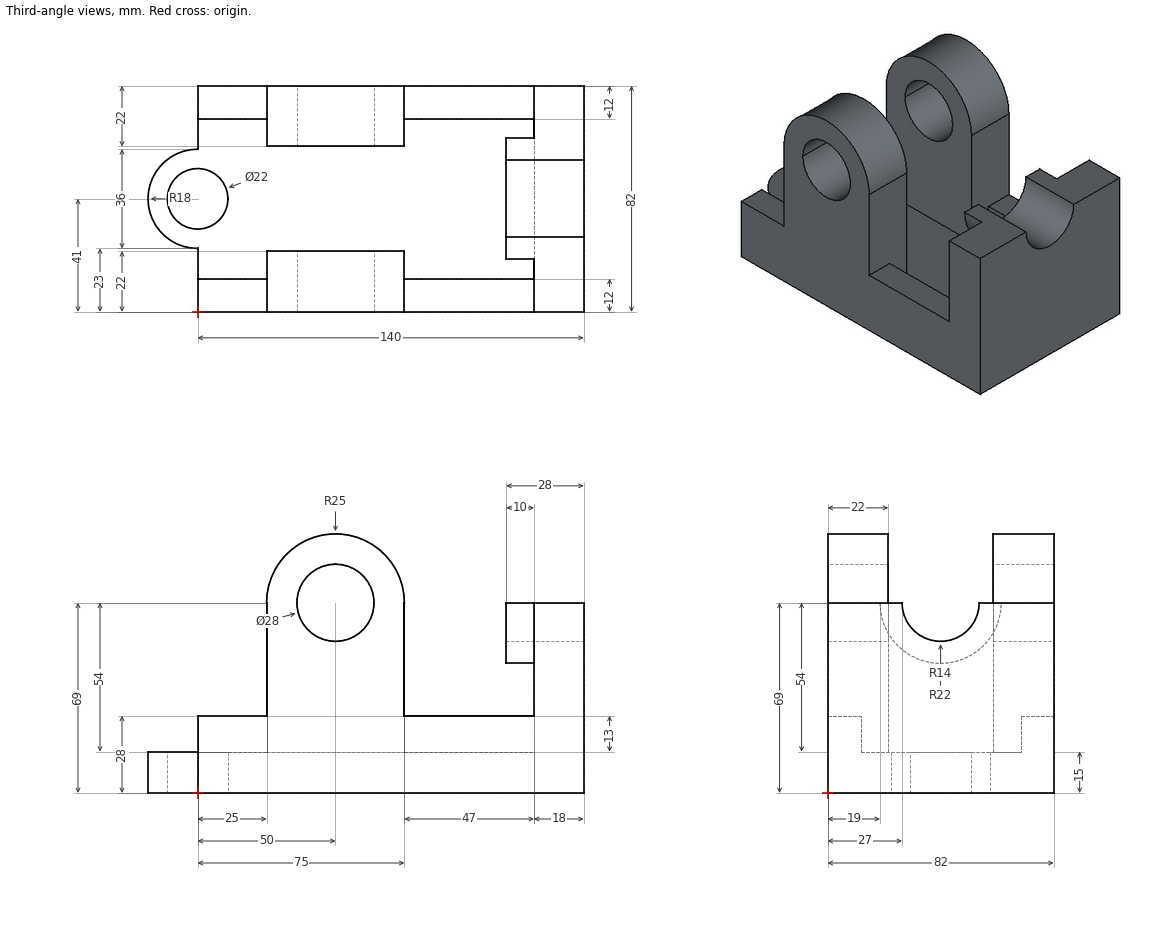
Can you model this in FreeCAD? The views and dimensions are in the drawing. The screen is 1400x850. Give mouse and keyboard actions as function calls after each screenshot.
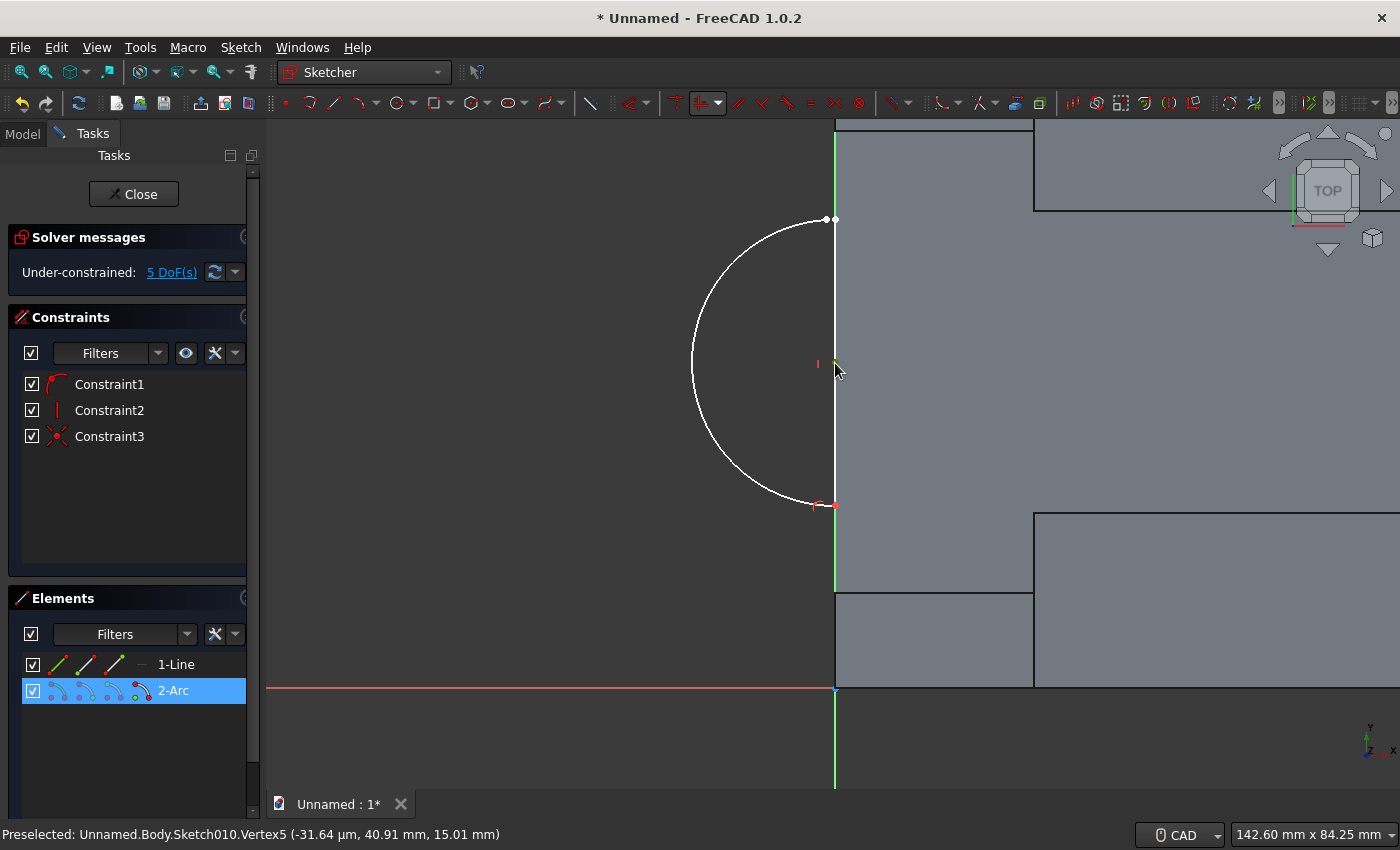
click(835, 629)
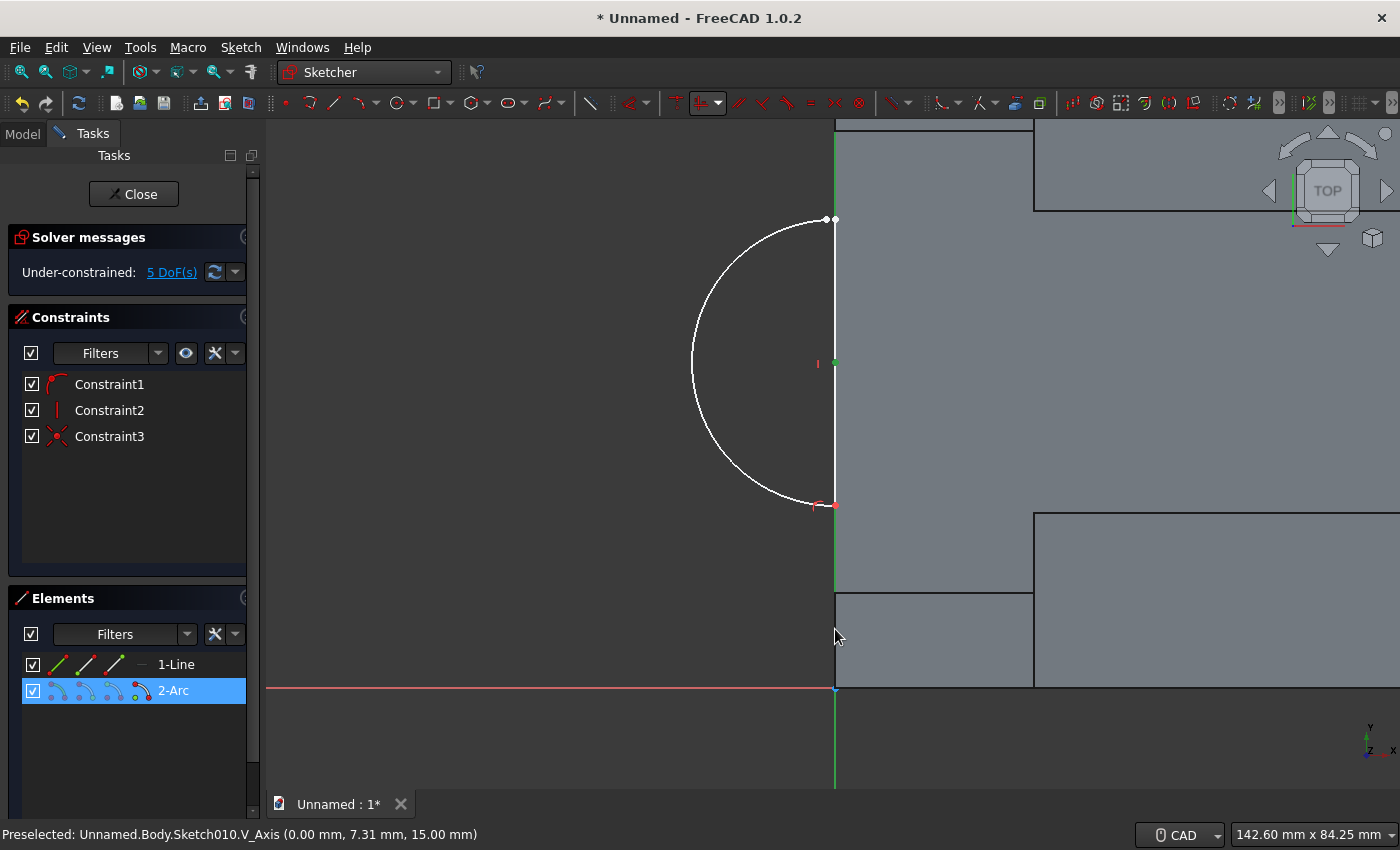
click(676, 104)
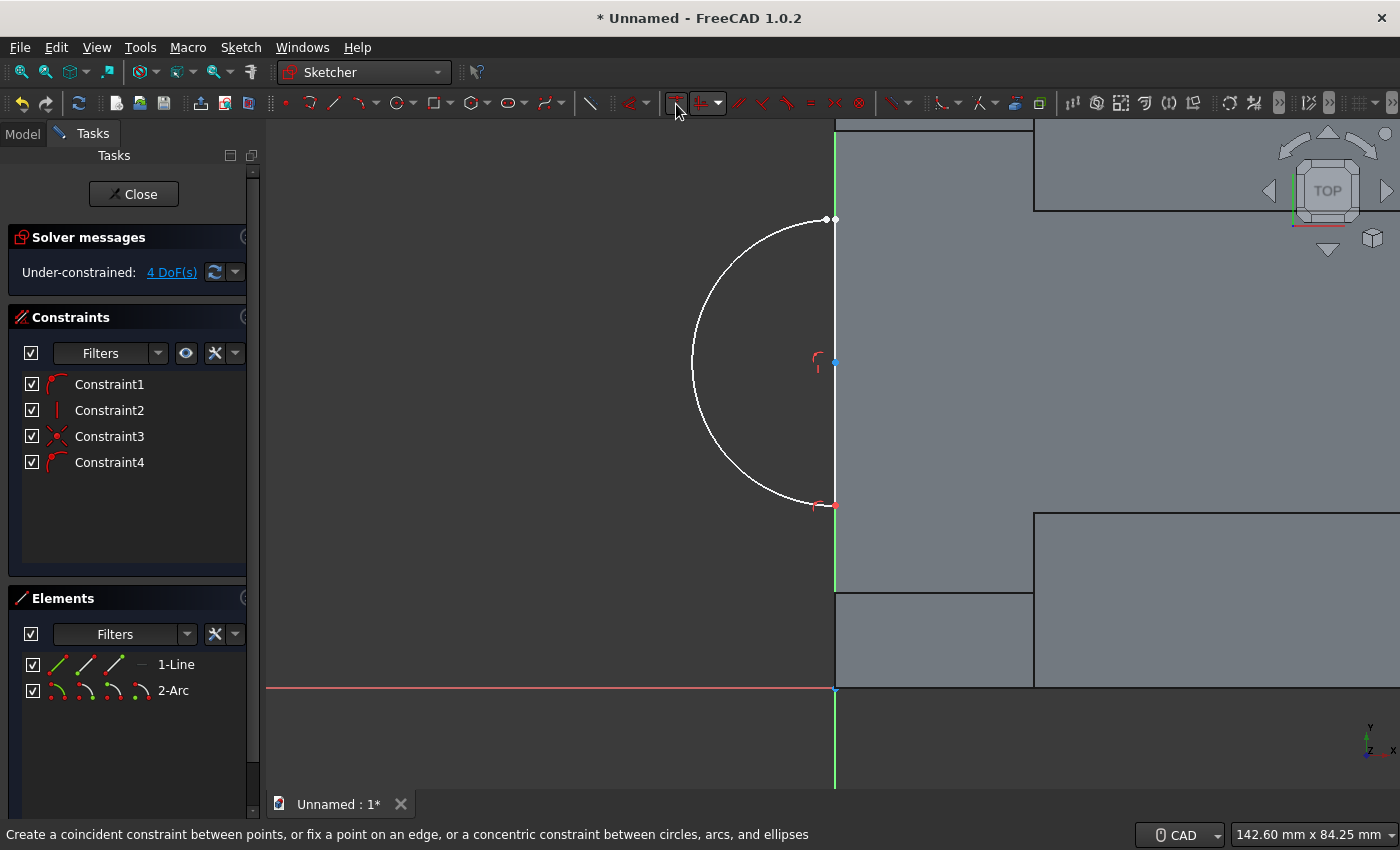
click(630, 104)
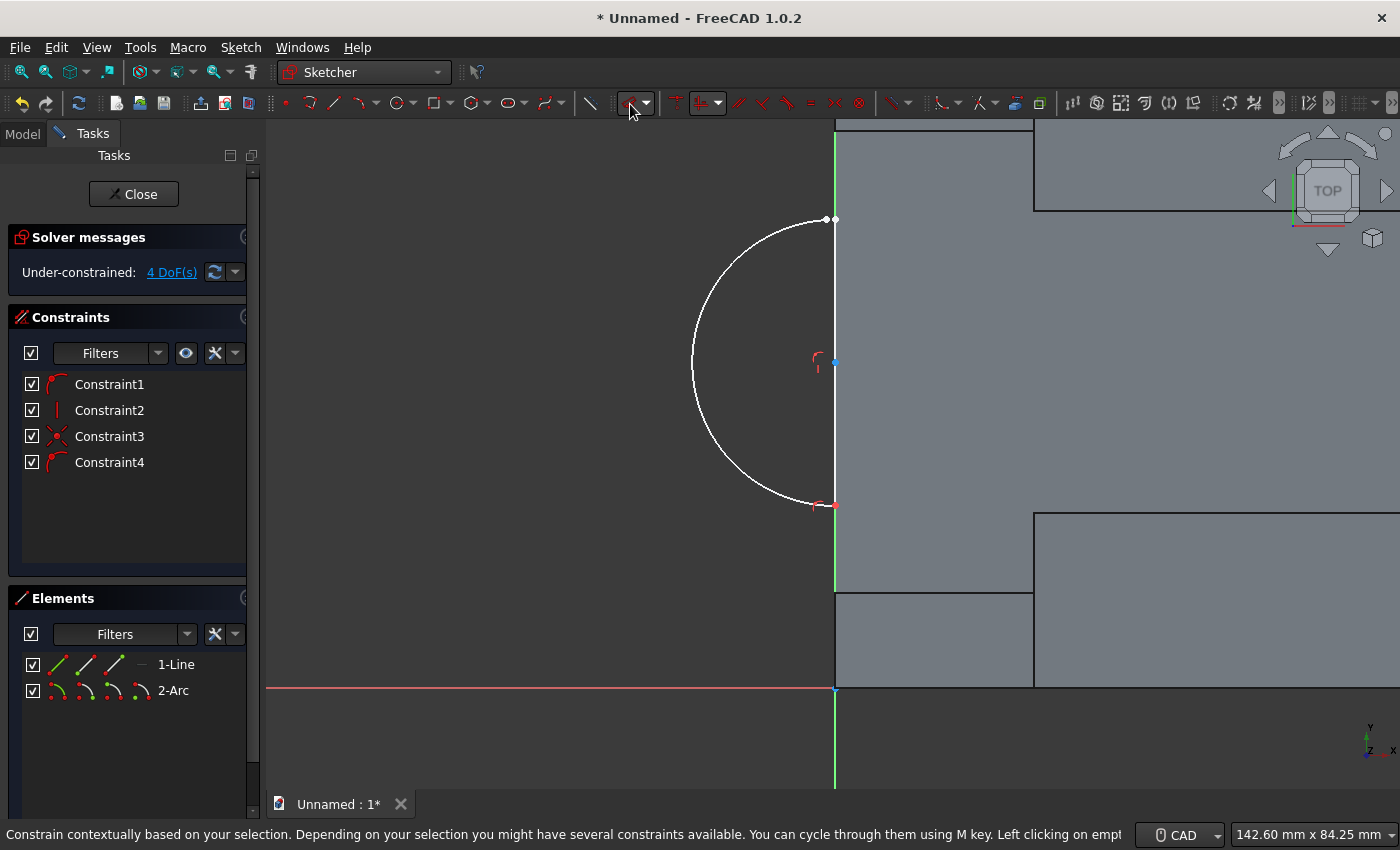
click(716, 284)
click(689, 266)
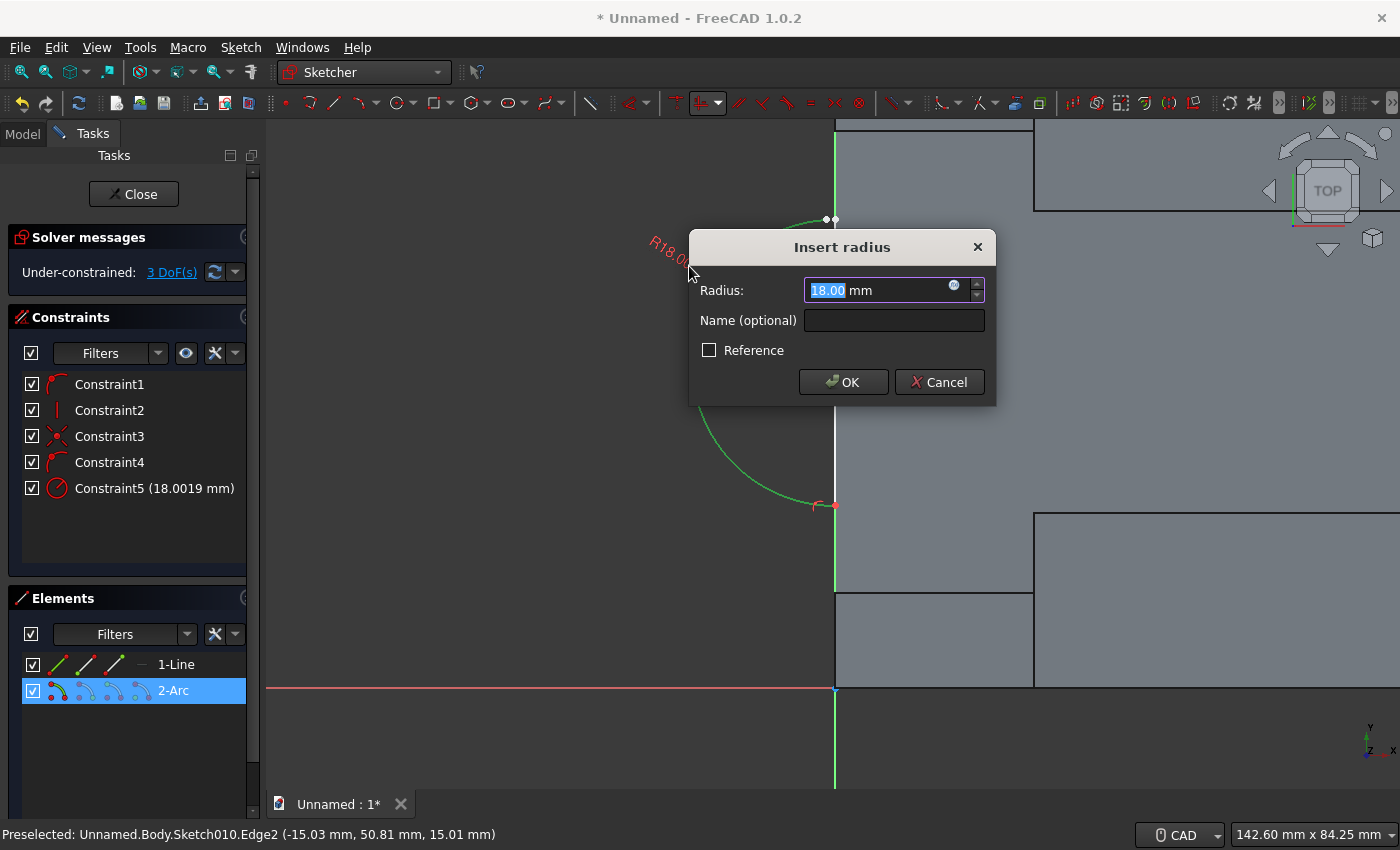
text(18)
key(Return)
key(Escape)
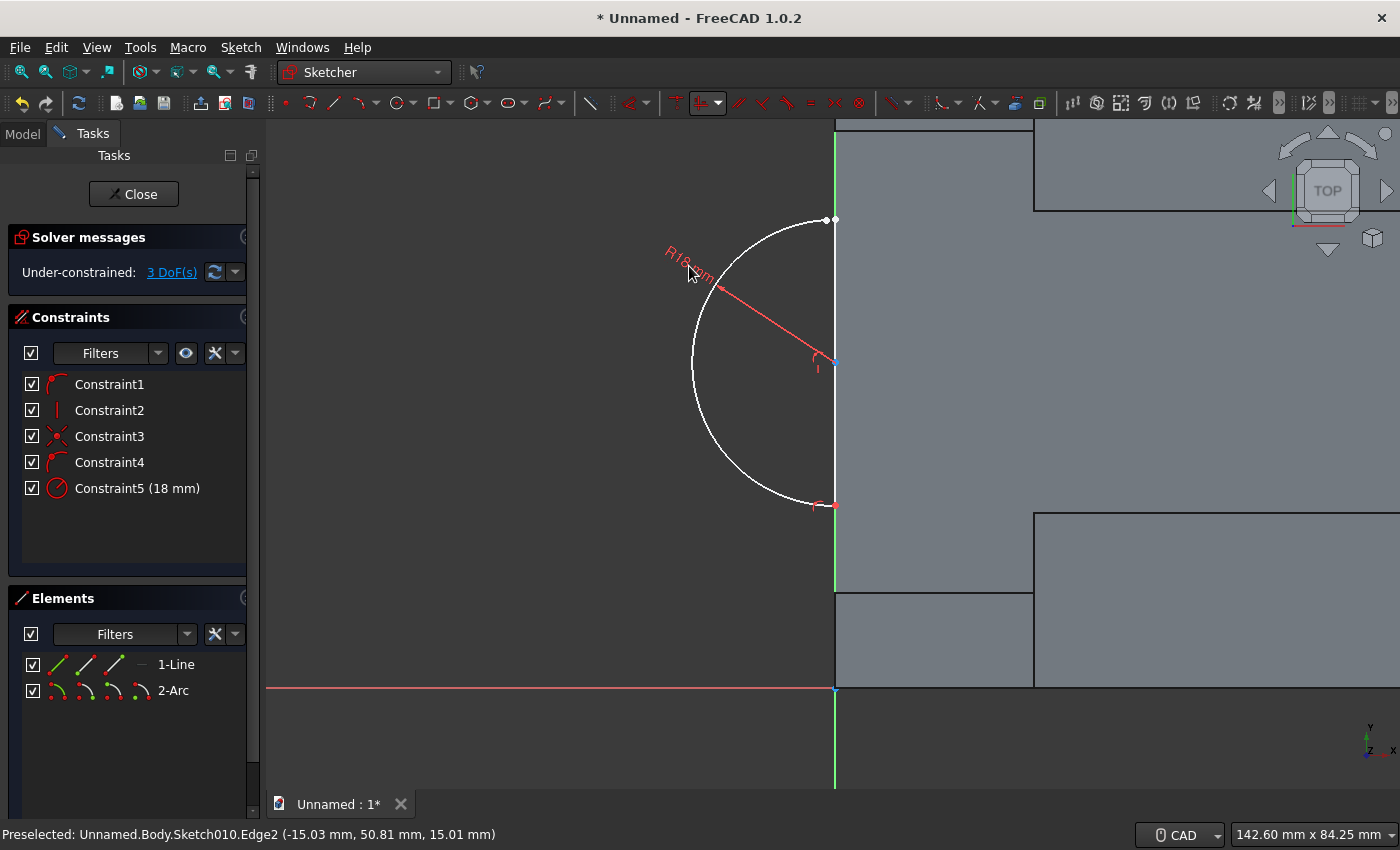
click(826, 220)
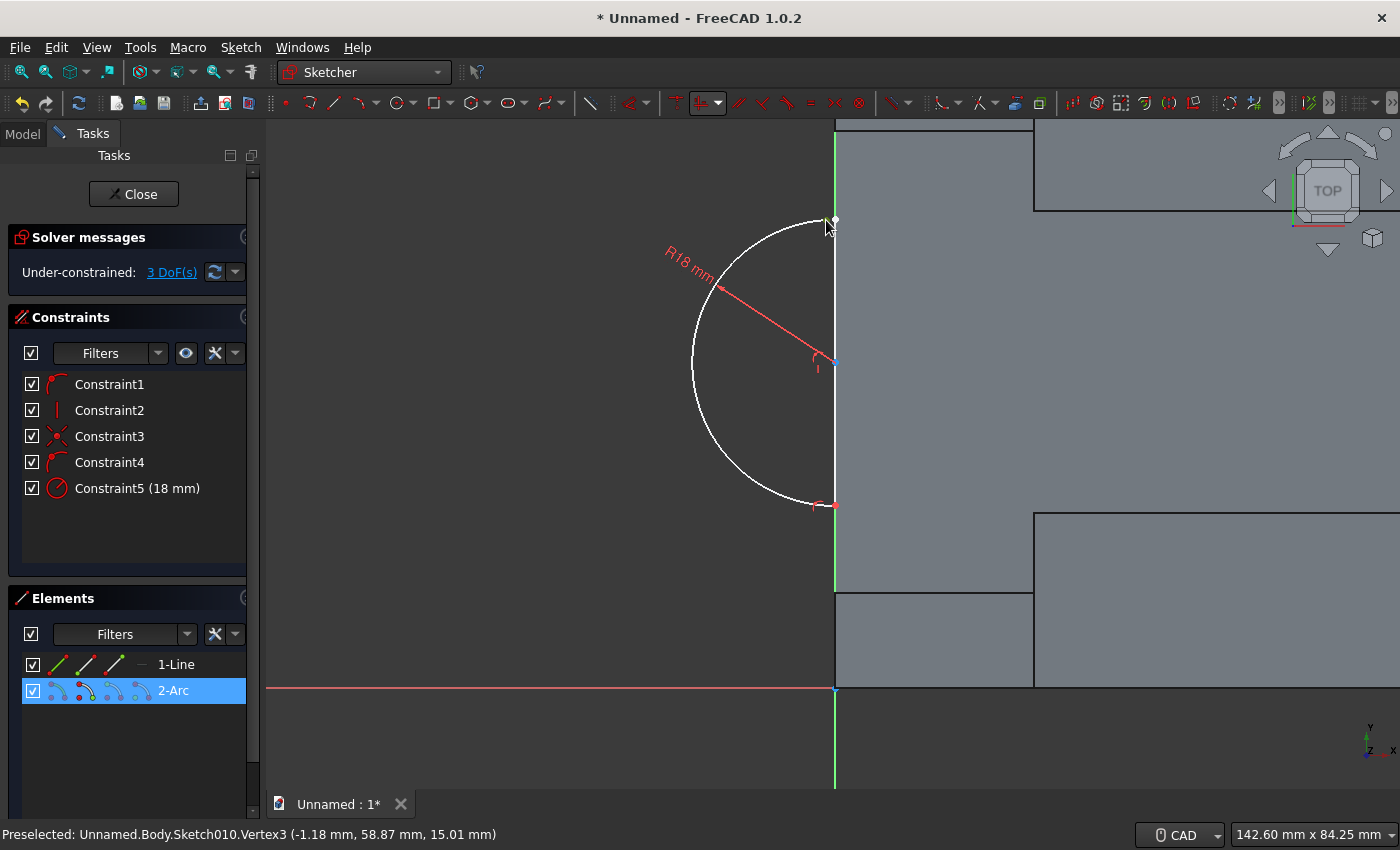
click(835, 629)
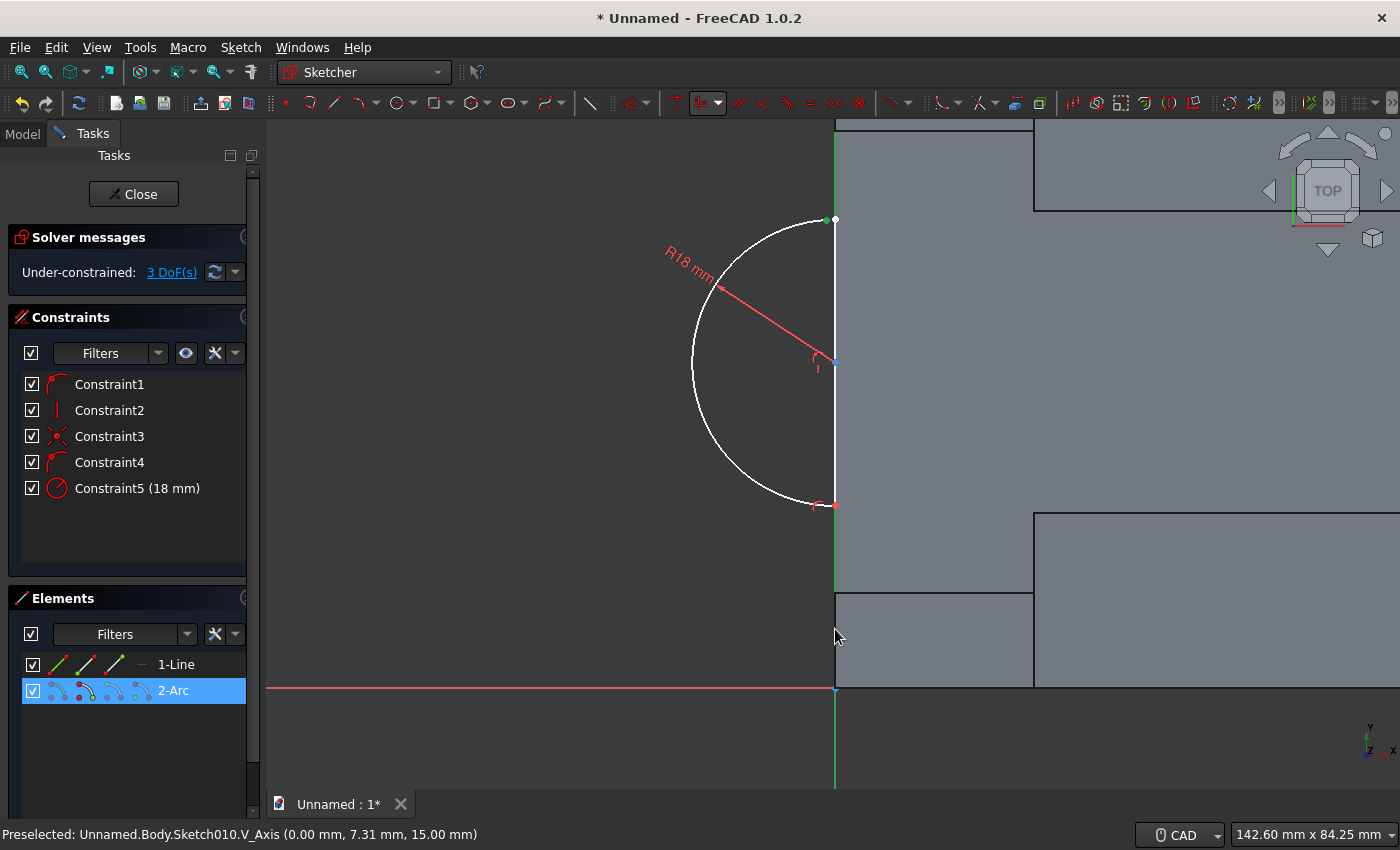
click(676, 104)